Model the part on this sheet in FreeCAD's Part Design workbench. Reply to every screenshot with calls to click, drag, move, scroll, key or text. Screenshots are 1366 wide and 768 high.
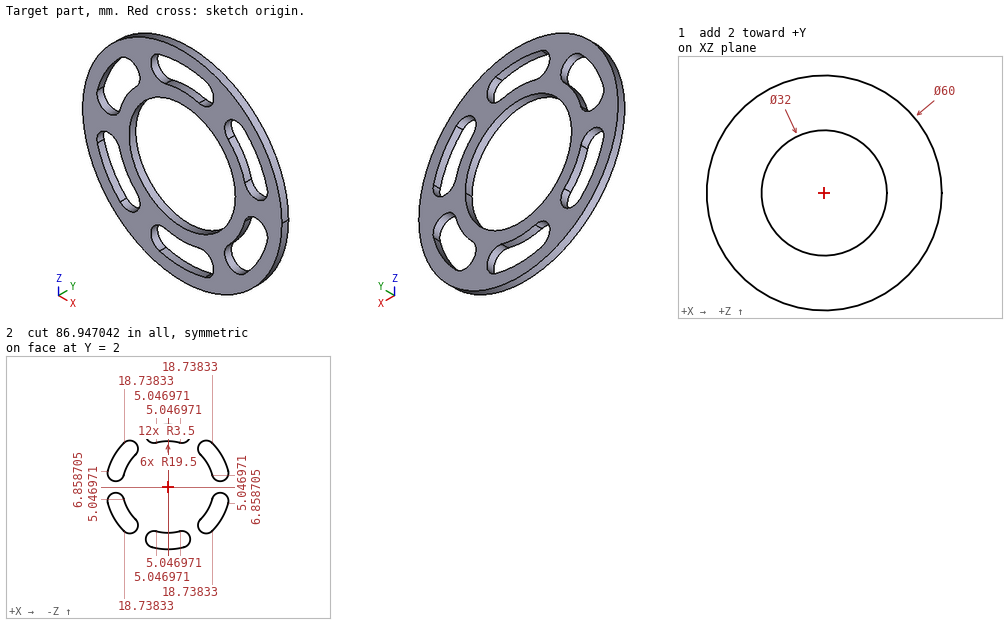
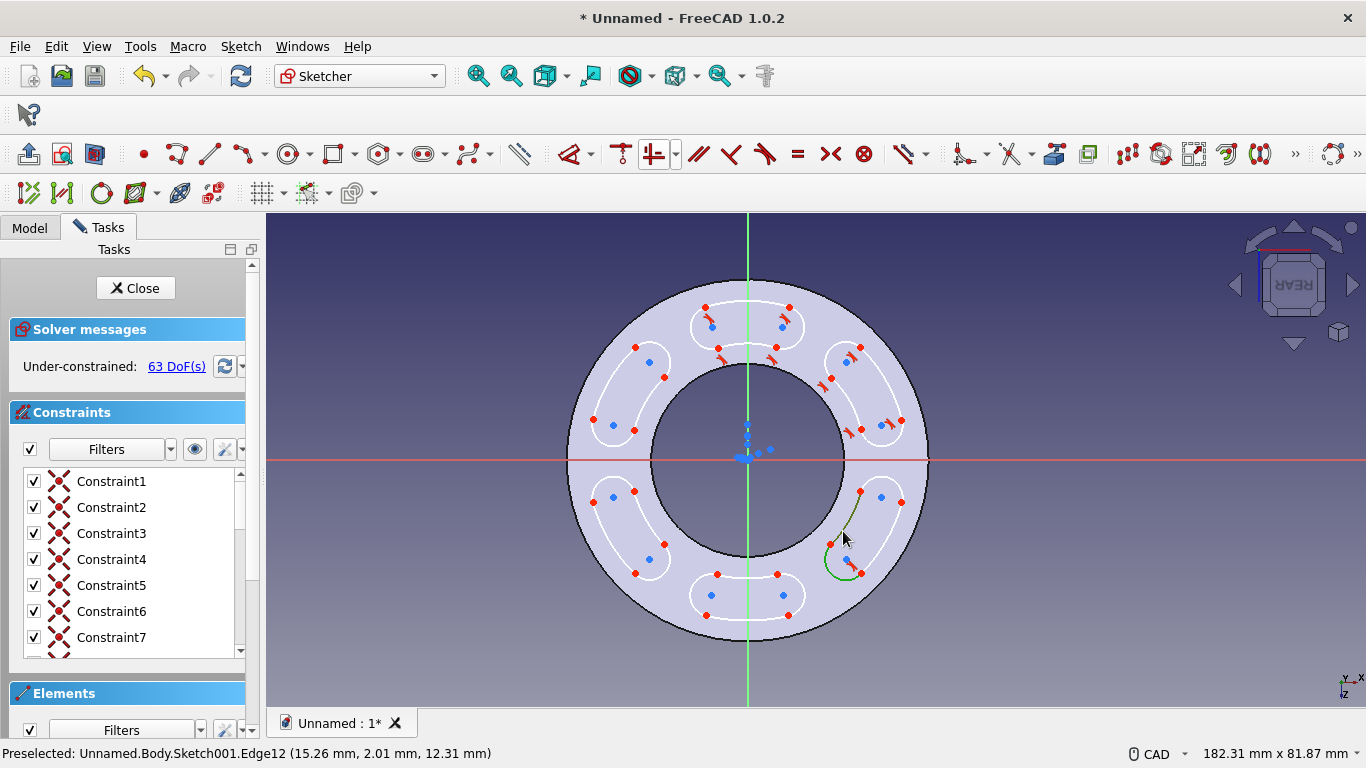
click(765, 154)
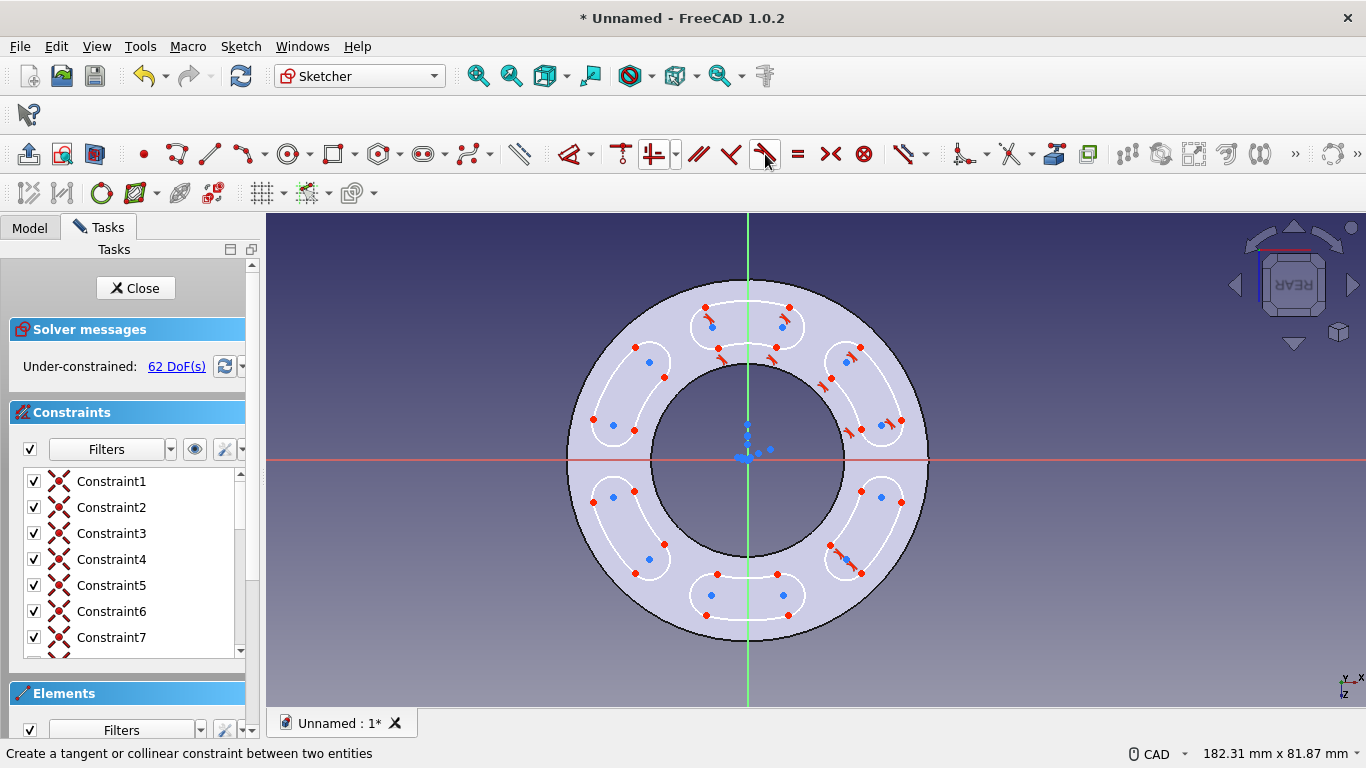
click(877, 555)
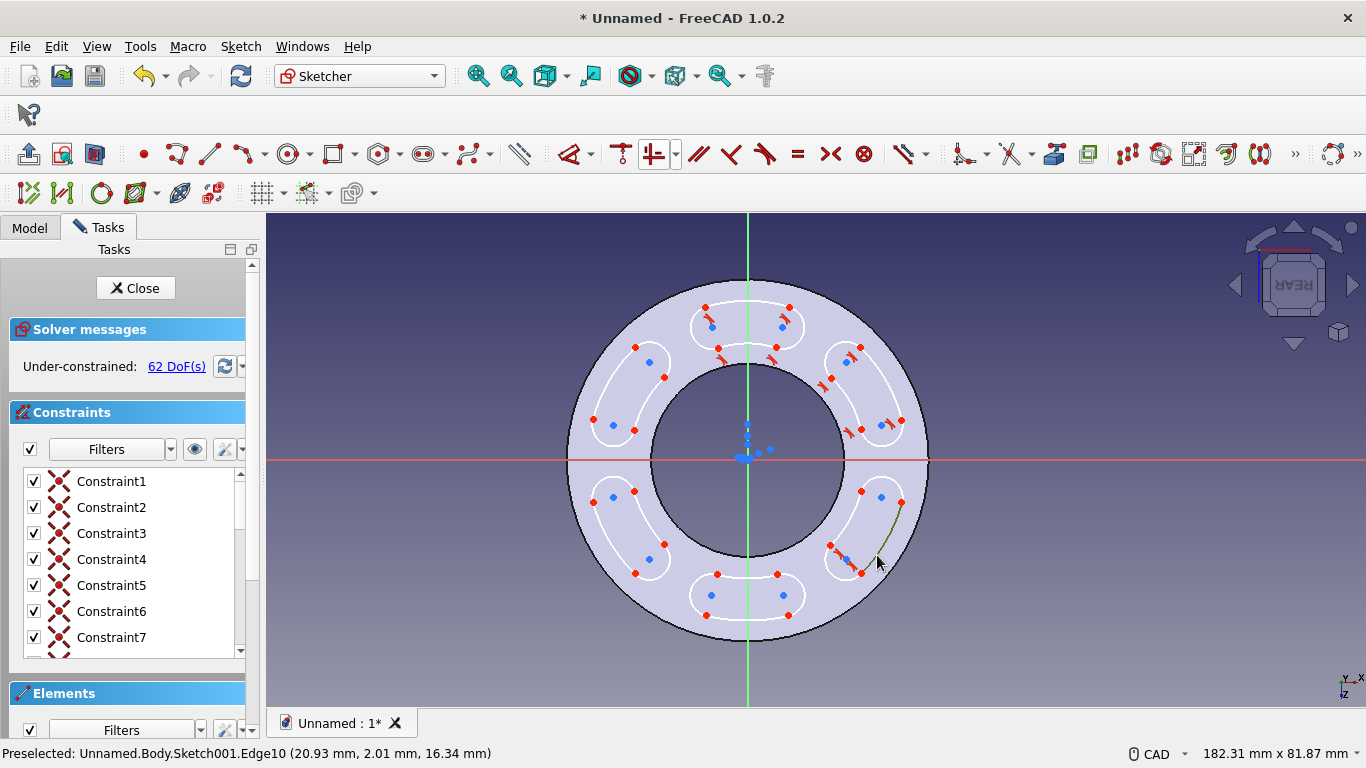
click(898, 484)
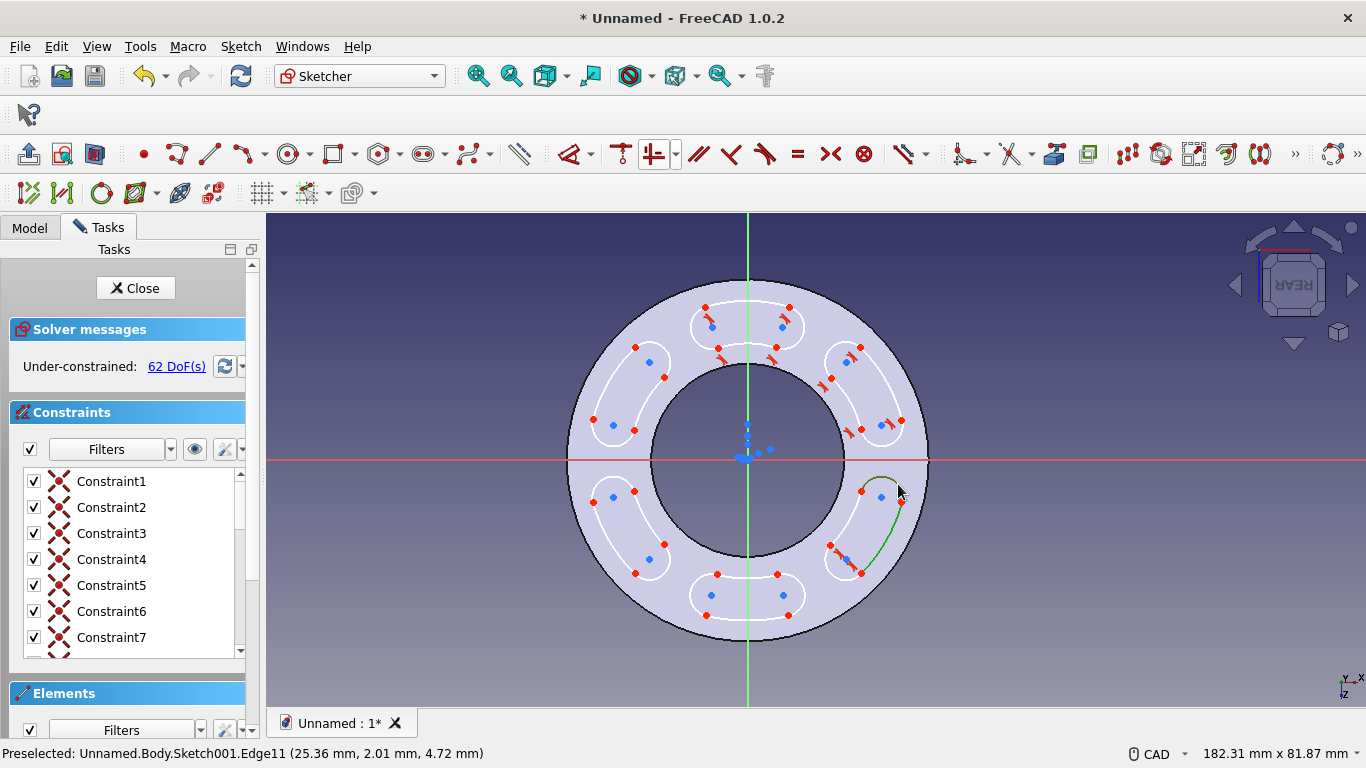
click(765, 154)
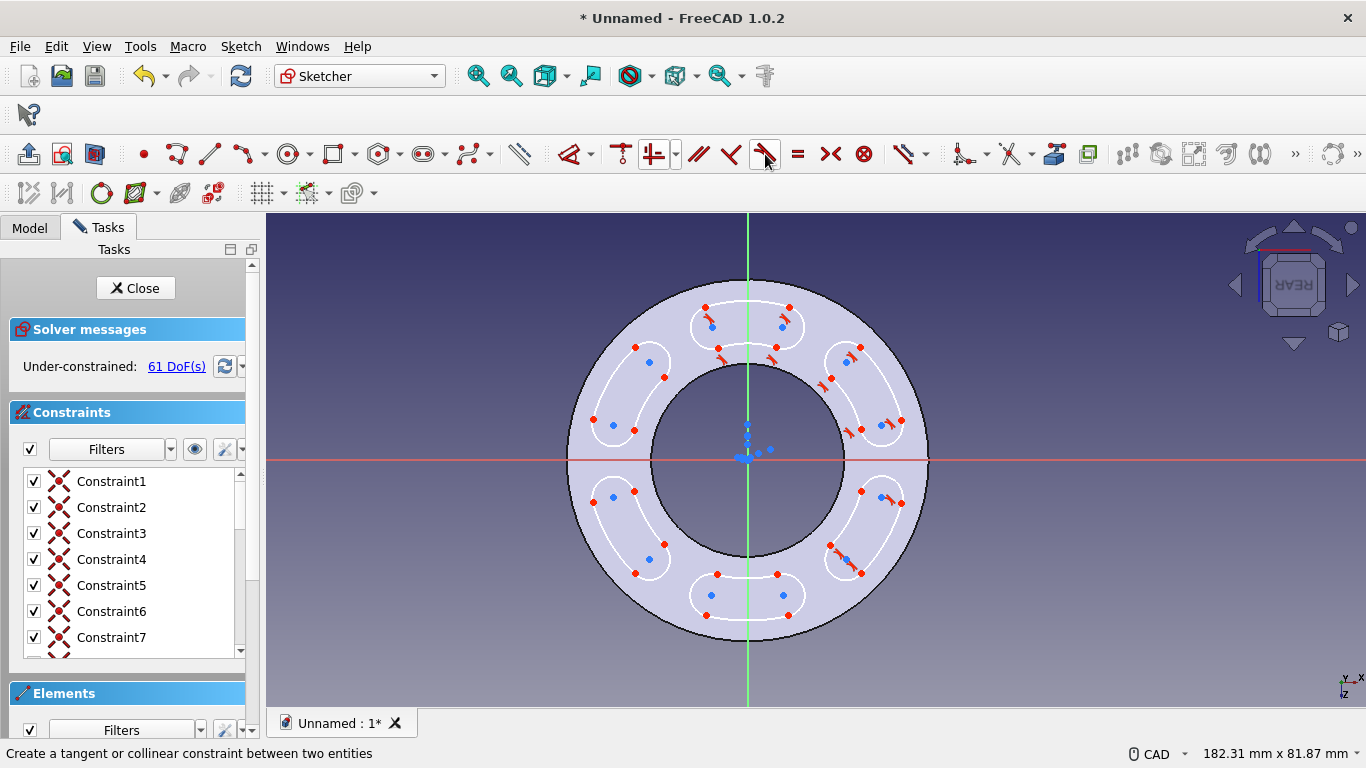
click(898, 484)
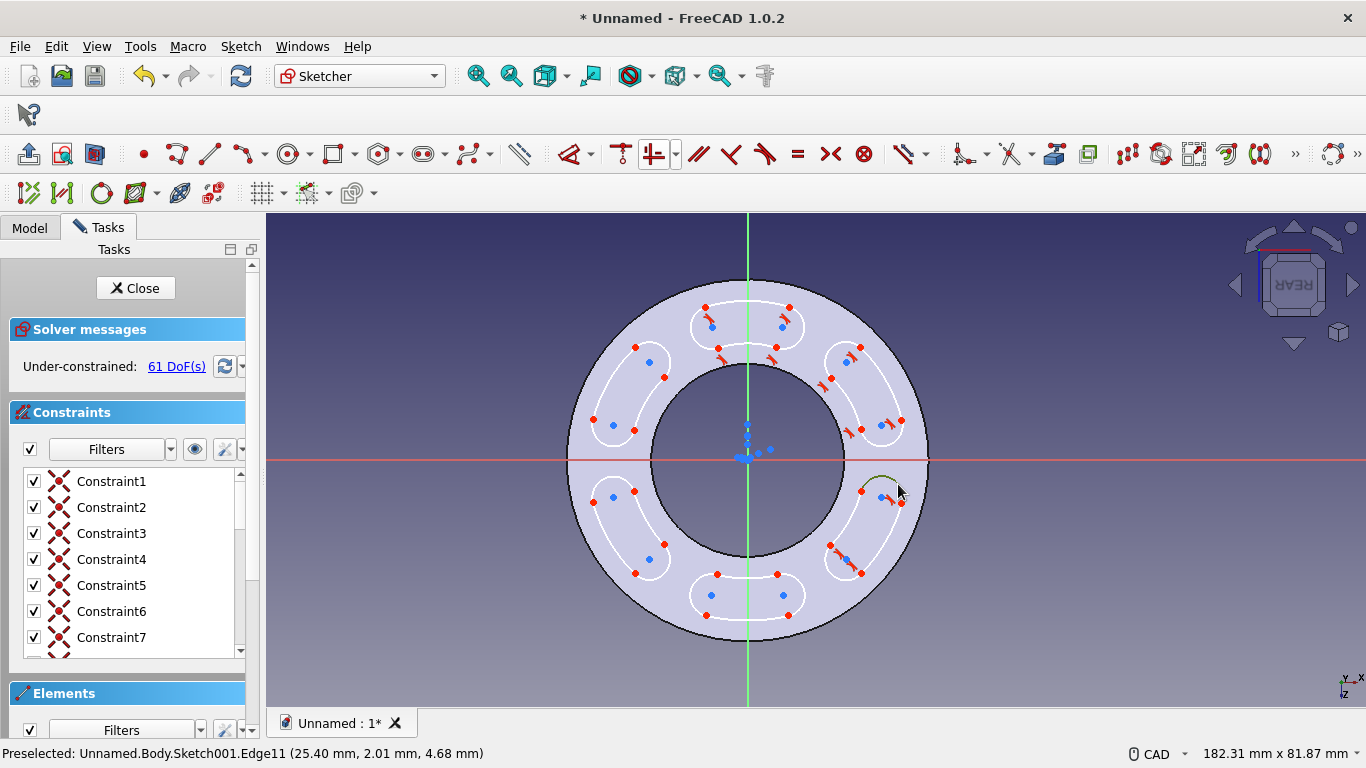
click(843, 531)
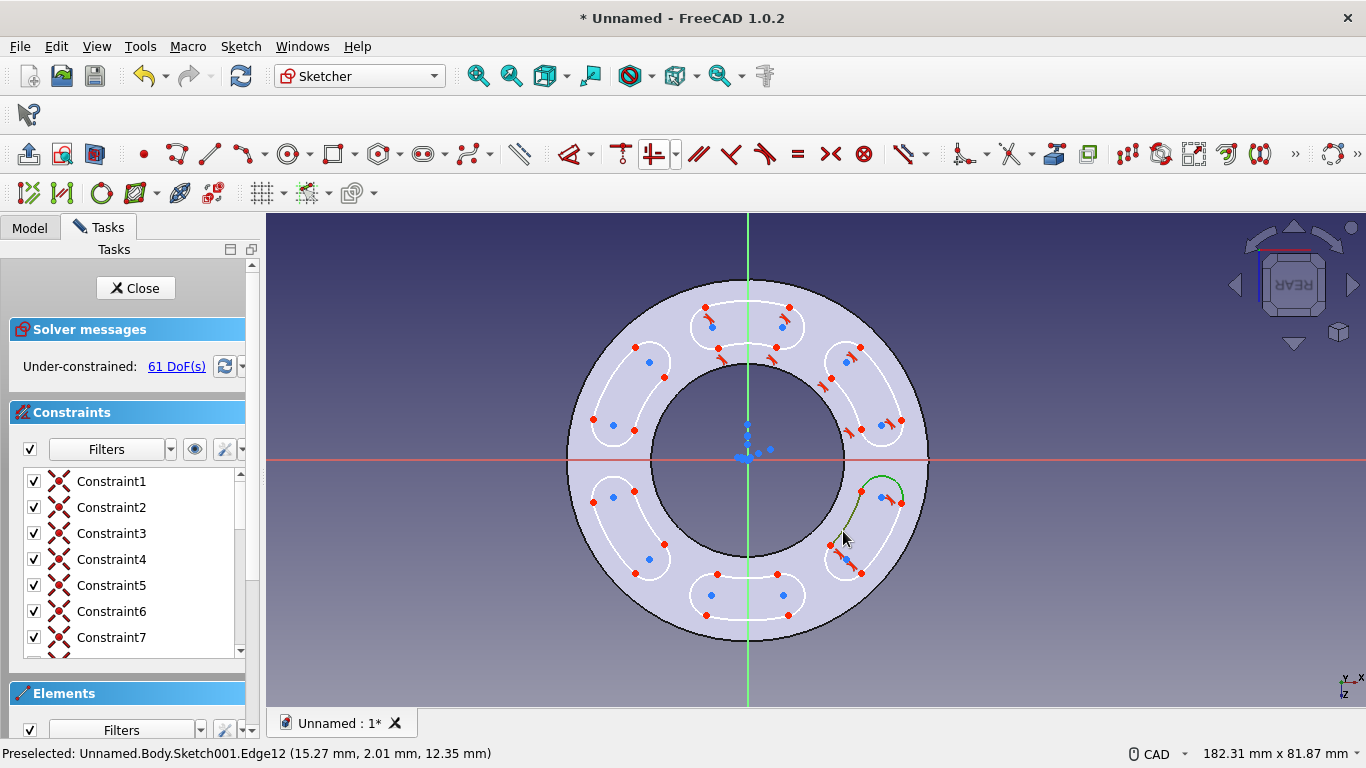
click(765, 154)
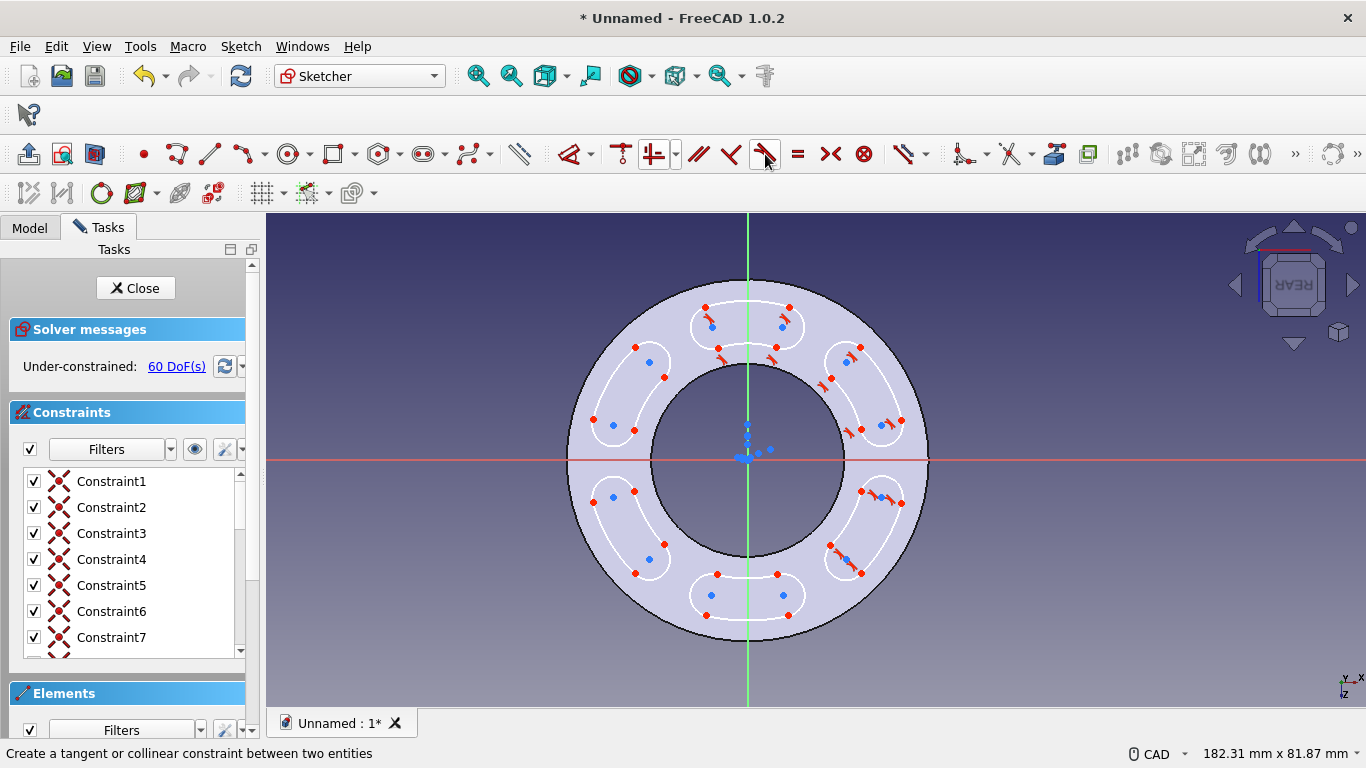
click(735, 578)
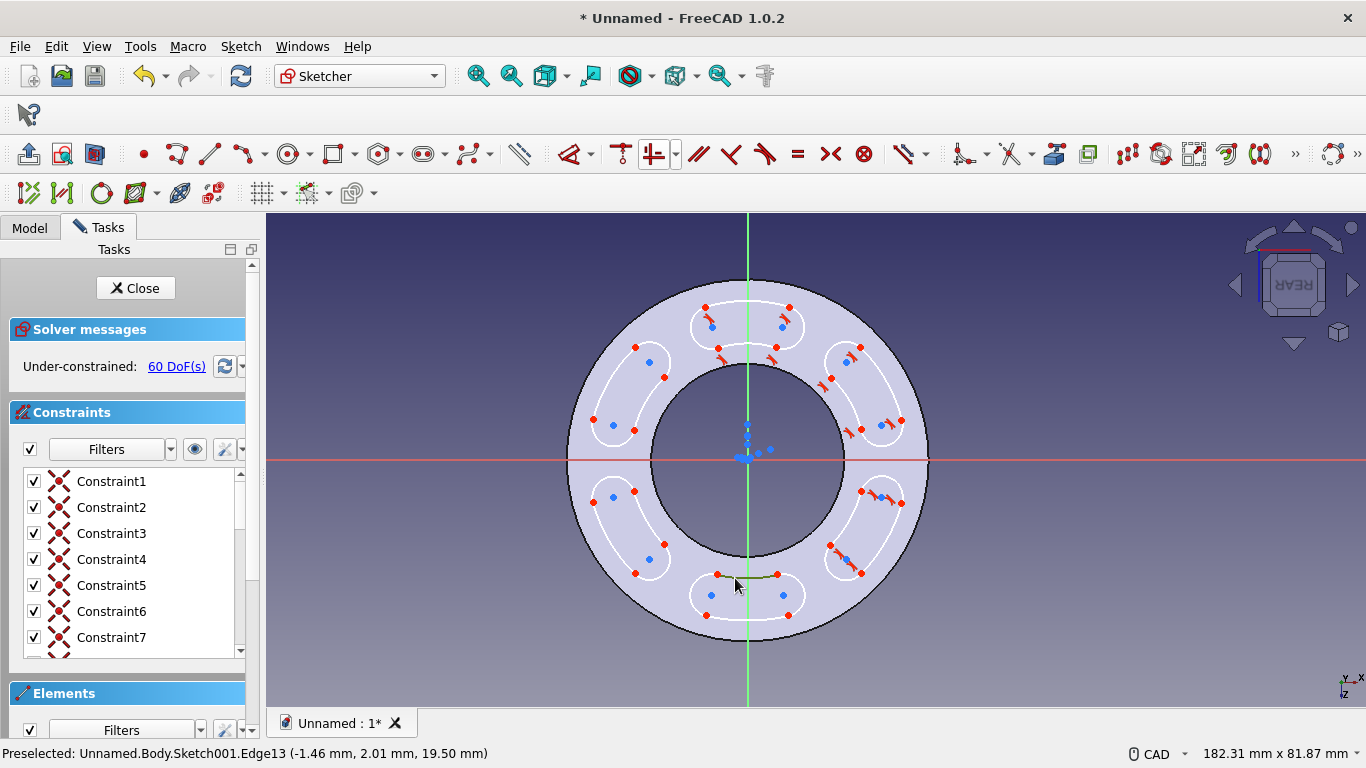
click(698, 579)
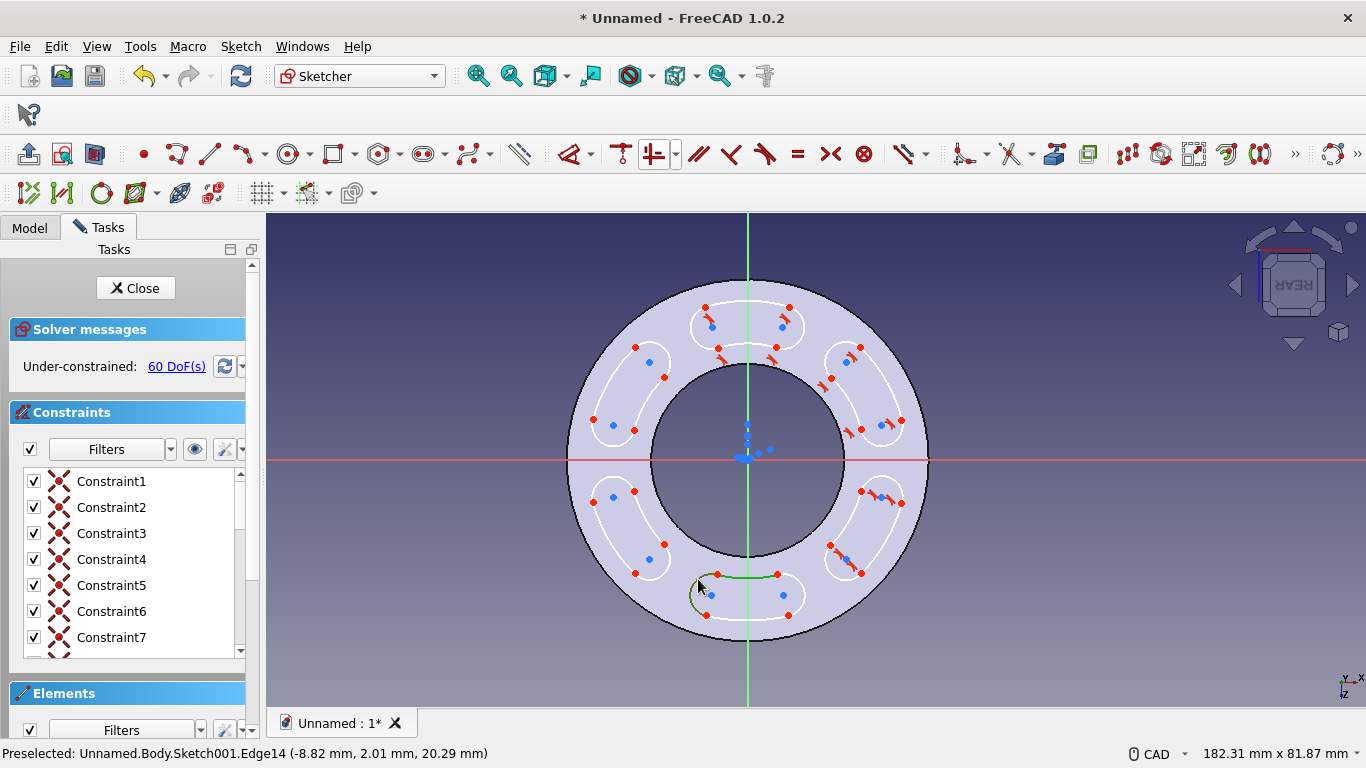
click(765, 154)